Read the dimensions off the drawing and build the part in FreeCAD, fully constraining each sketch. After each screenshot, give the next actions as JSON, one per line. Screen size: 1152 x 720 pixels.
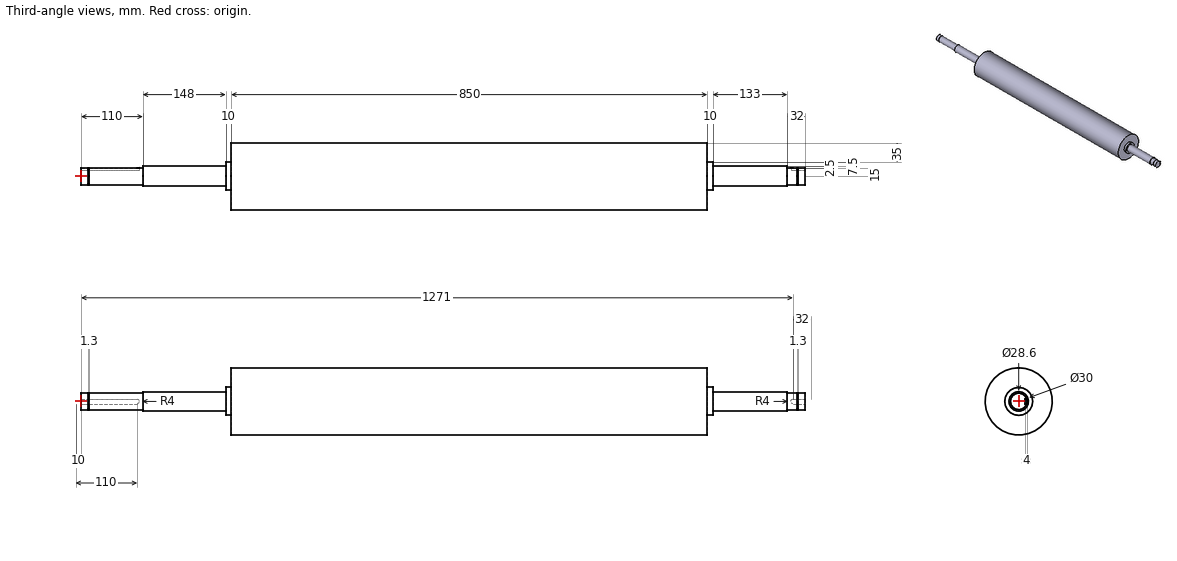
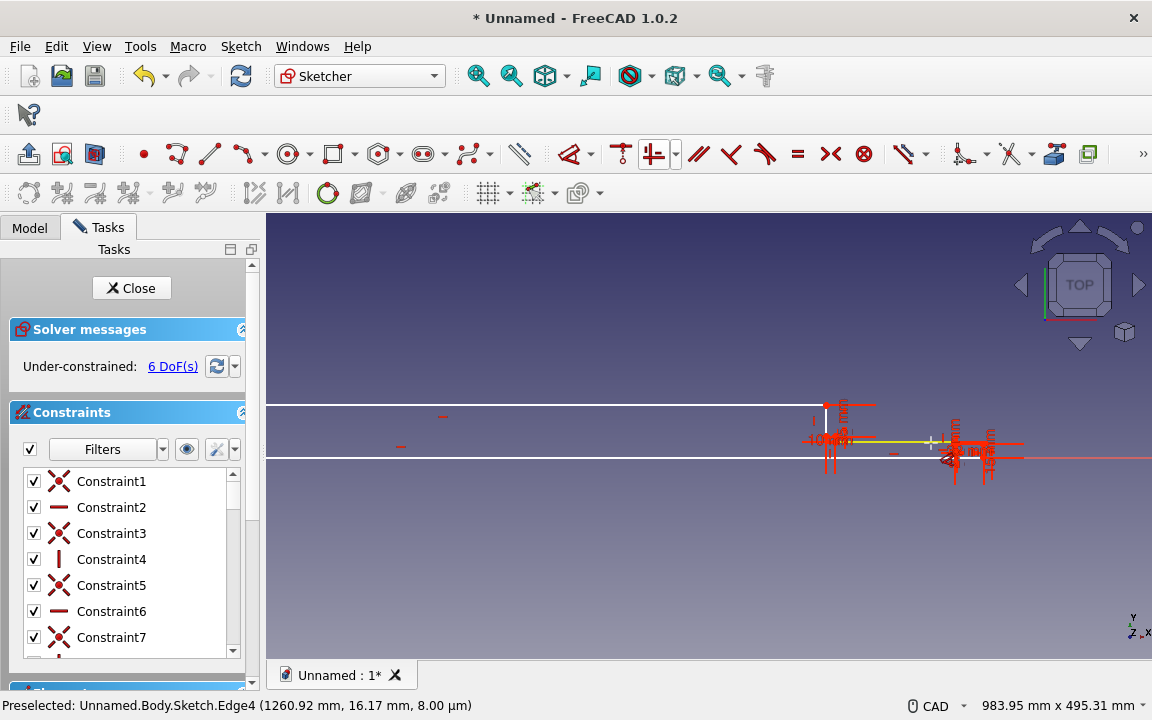
{"action": "left_click", "coordinate": [931, 442]}
{"action": "left_click", "coordinate": [895, 476]}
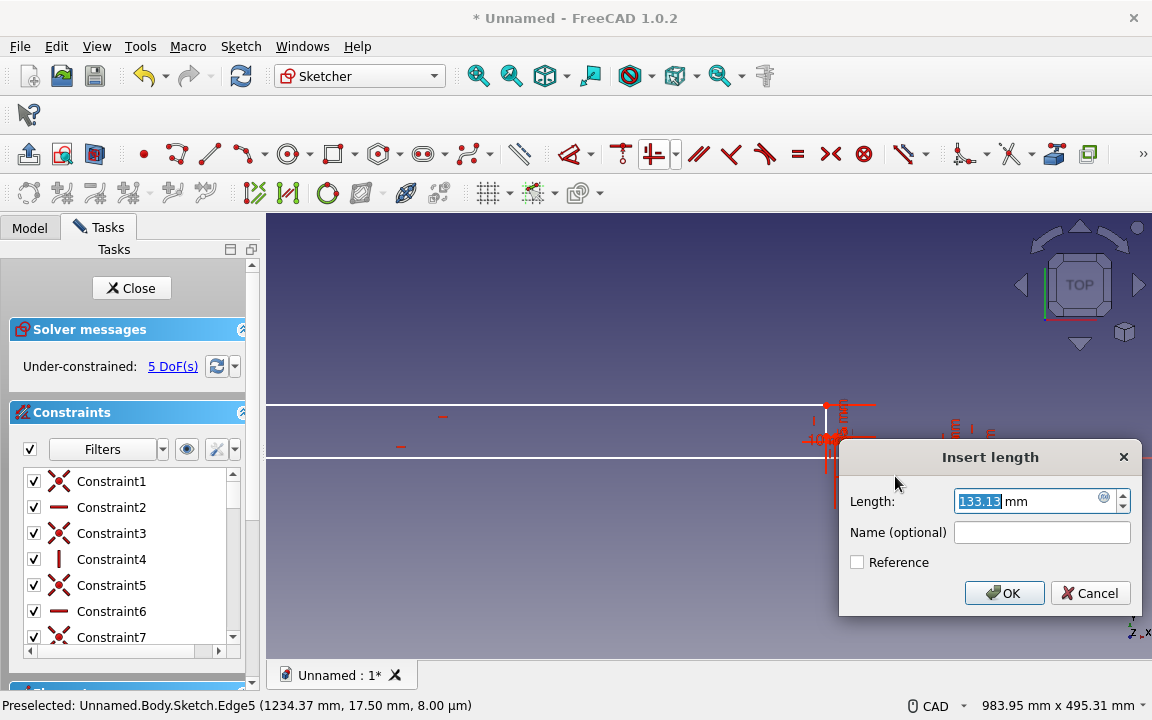
{"action": "type", "text": "133"}
{"action": "key", "text": "Return"}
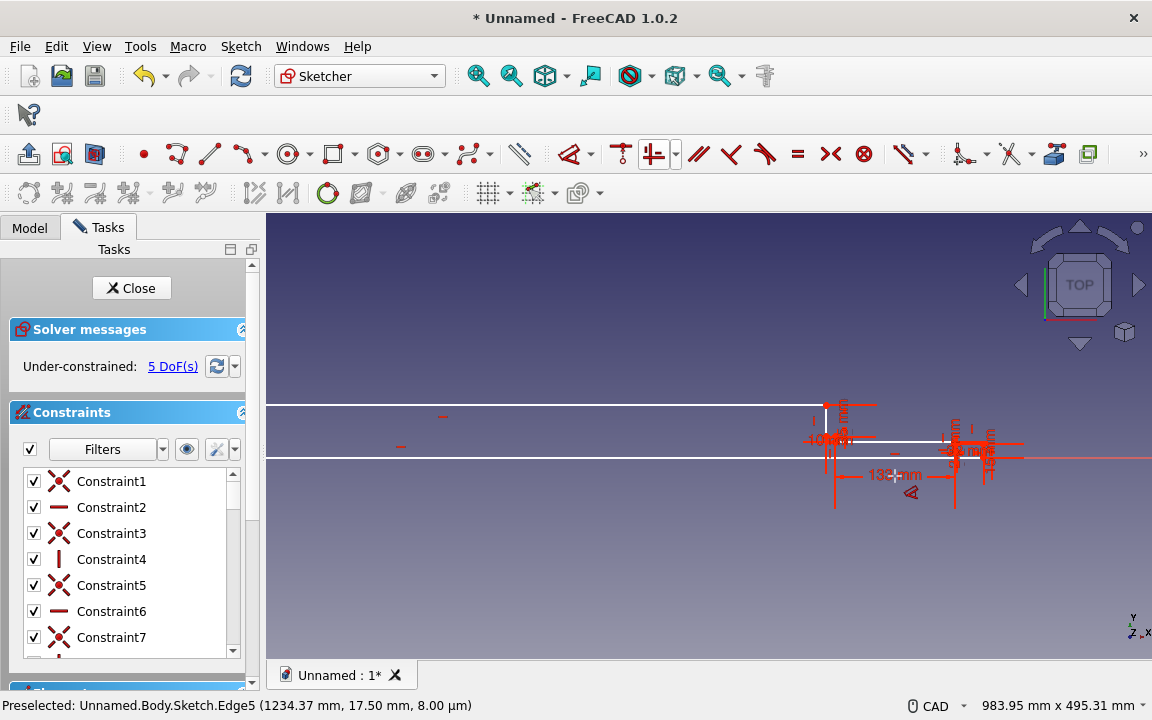
{"action": "scroll", "coordinate": [835, 439], "scroll_direction": "up", "scroll_amount": 9}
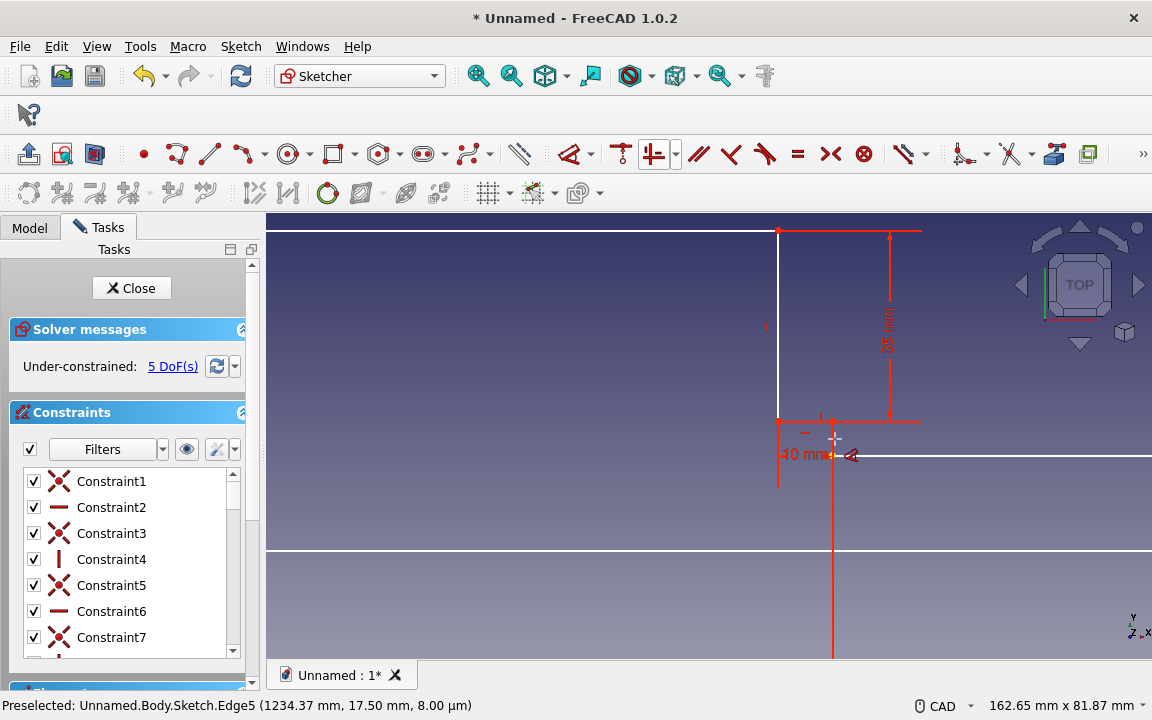
{"action": "left_click", "coordinate": [833, 439]}
{"action": "left_click", "coordinate": [867, 427]}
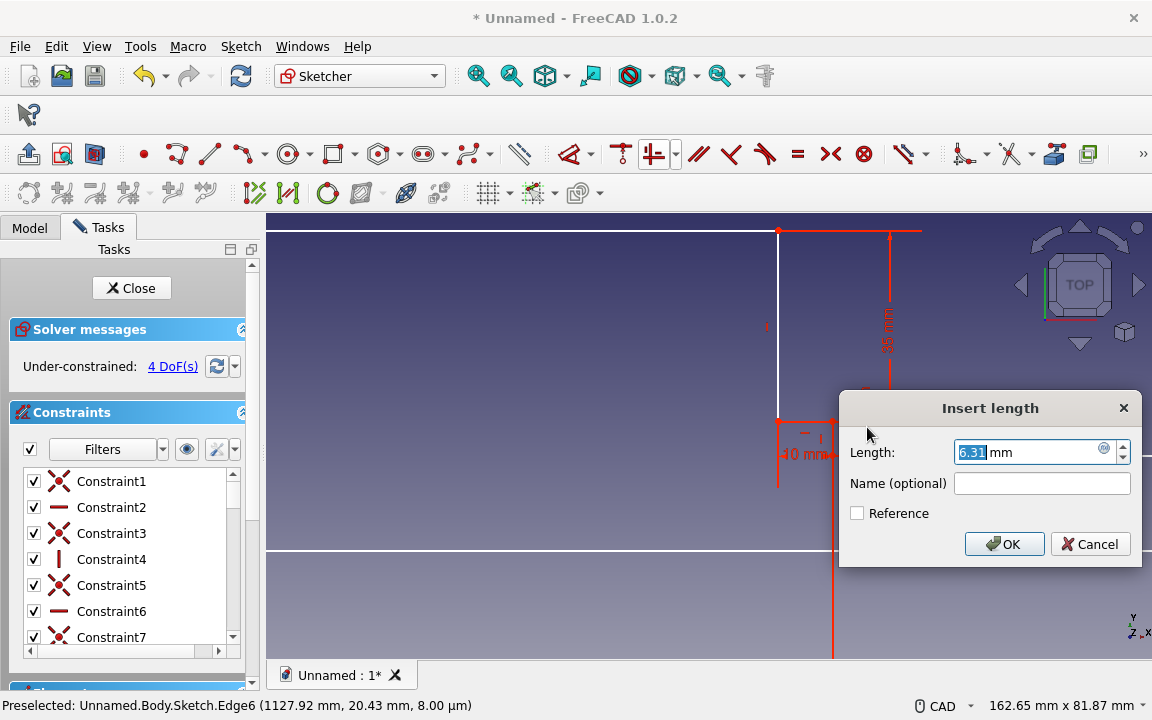
{"action": "type", "text": "7.5"}
{"action": "key", "text": "Return"}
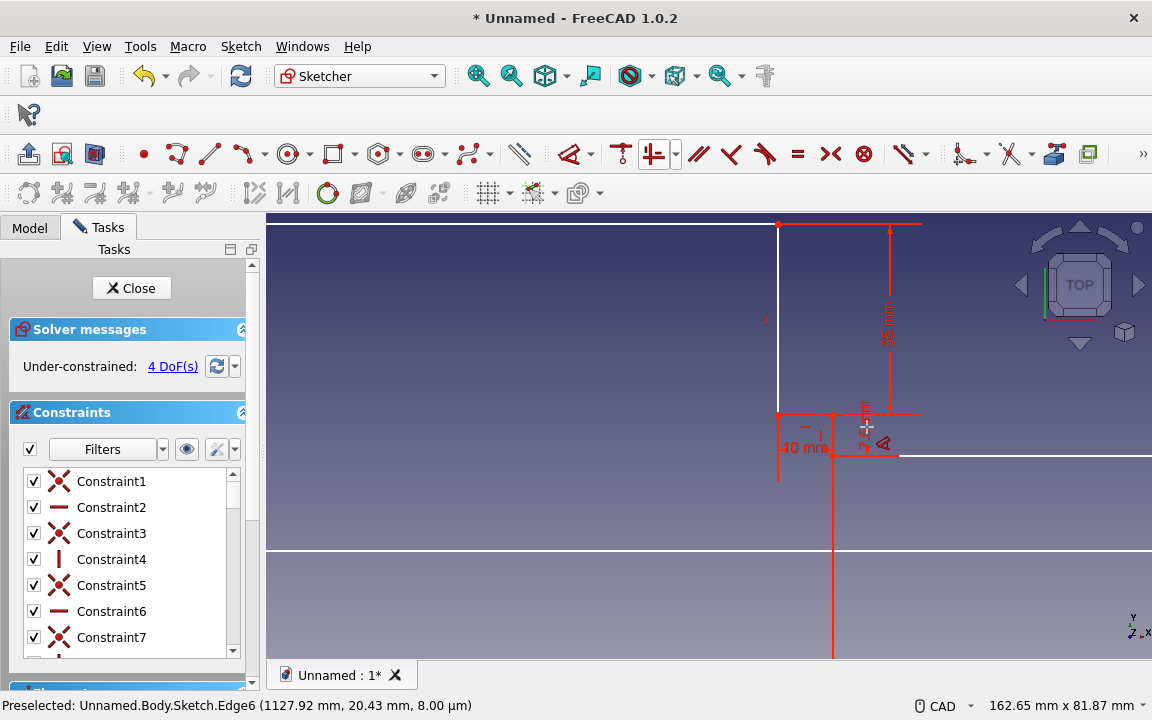
{"action": "scroll", "coordinate": [835, 440], "scroll_direction": "down", "scroll_amount": 13}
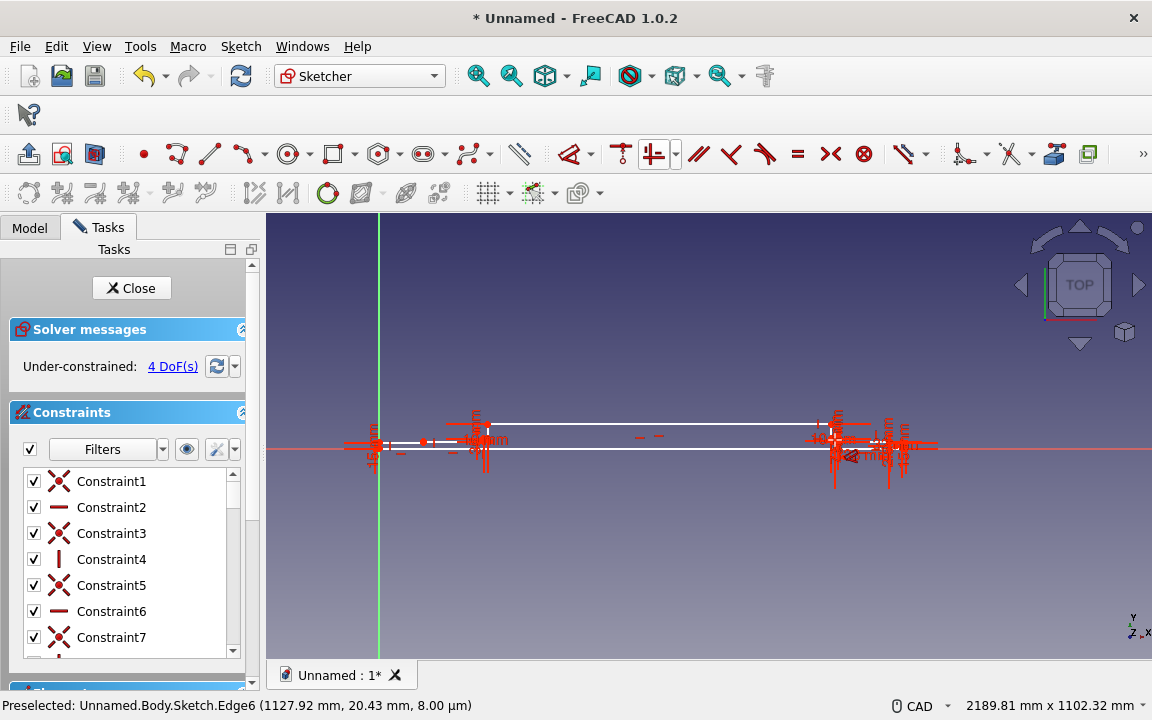
{"action": "left_click", "coordinate": [728, 424]}
{"action": "left_click", "coordinate": [660, 390]}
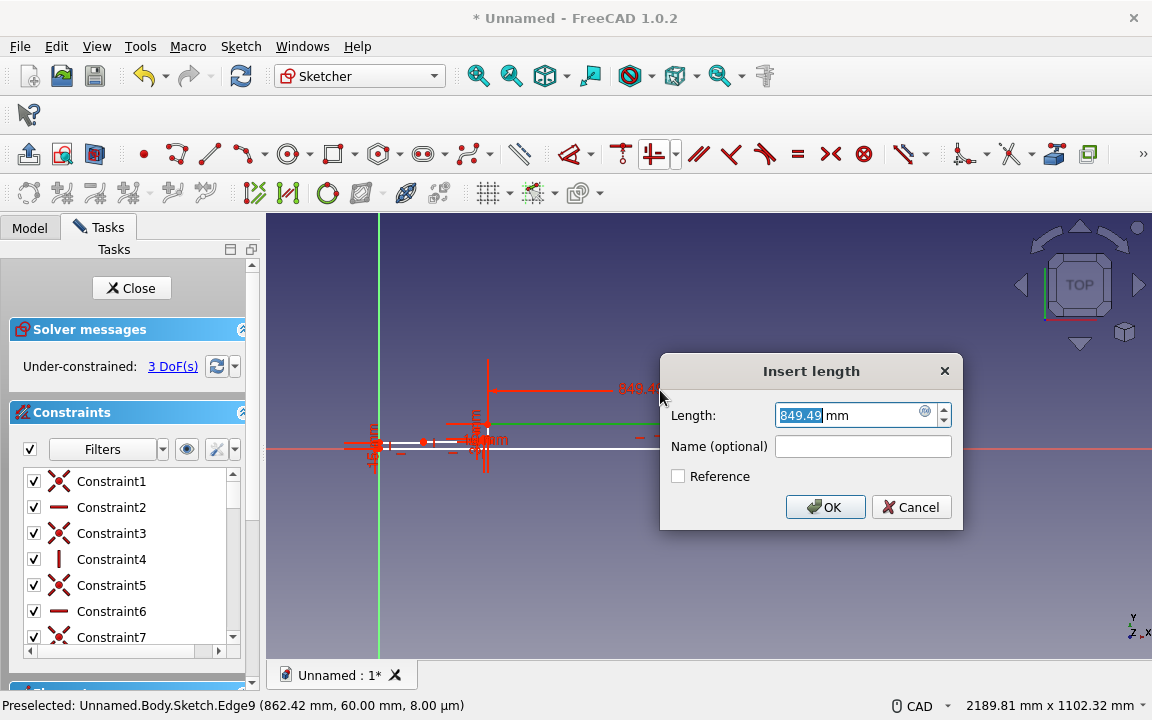
{"action": "type", "text": "850"}
{"action": "key", "text": "Return"}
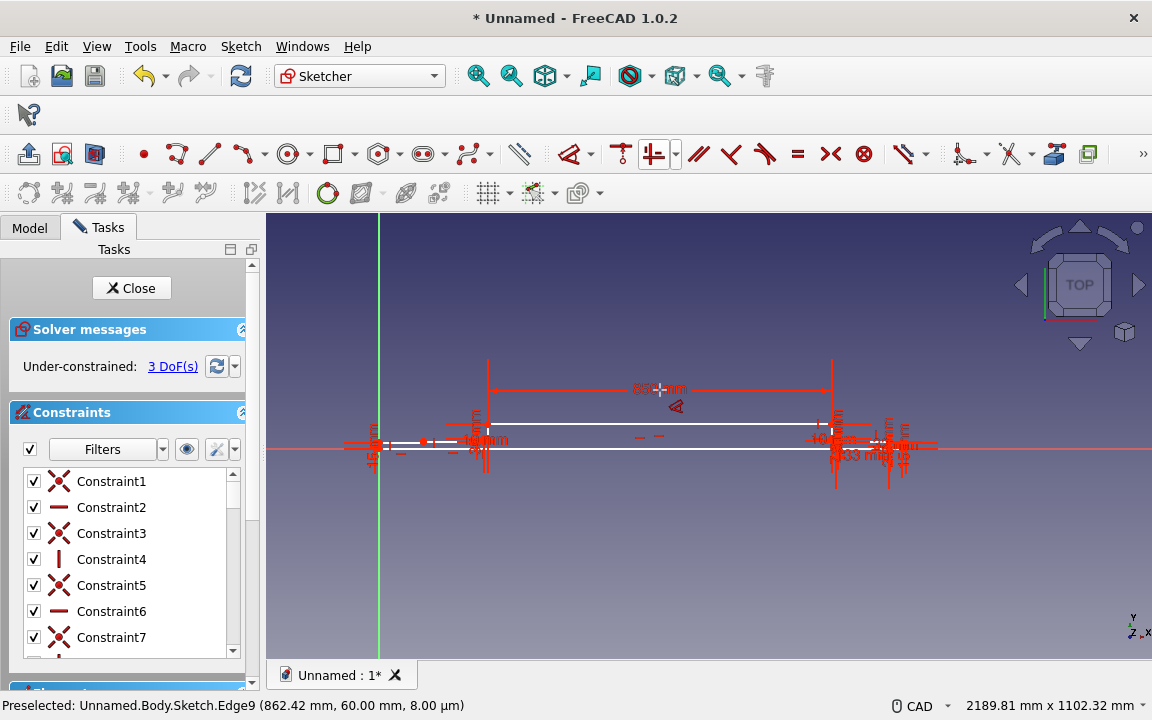
{"action": "scroll", "coordinate": [484, 440], "scroll_direction": "up", "scroll_amount": 13}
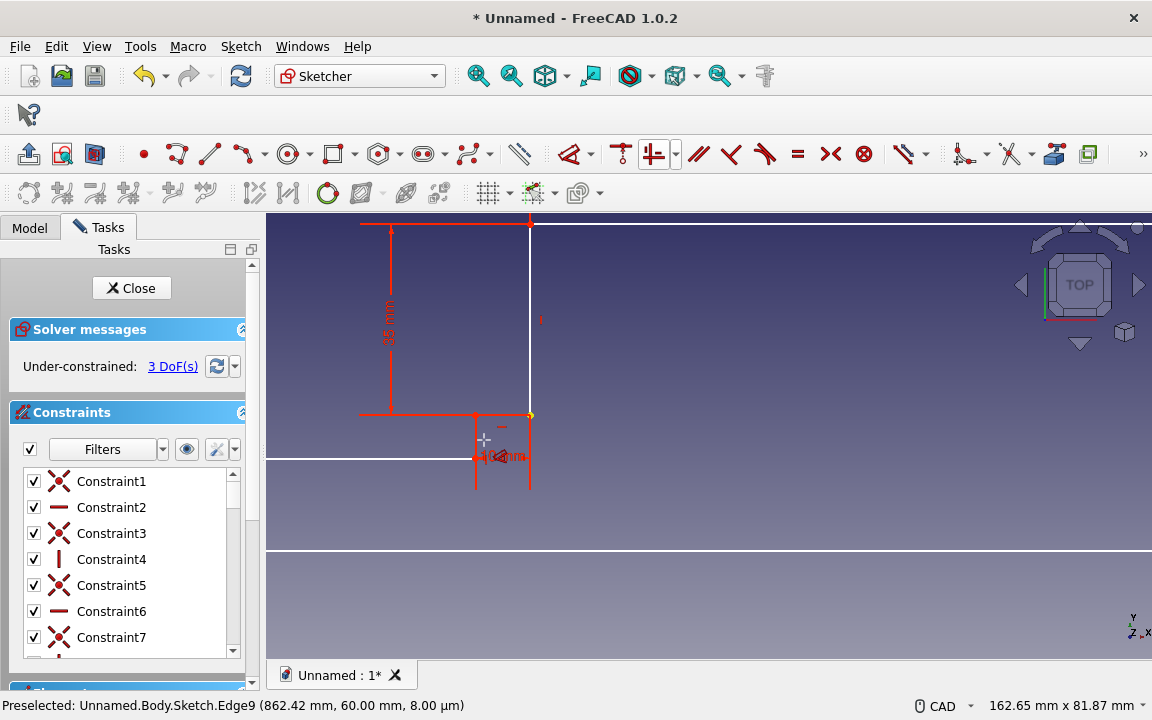
{"action": "left_click", "coordinate": [476, 437]}
{"action": "left_click", "coordinate": [442, 437]}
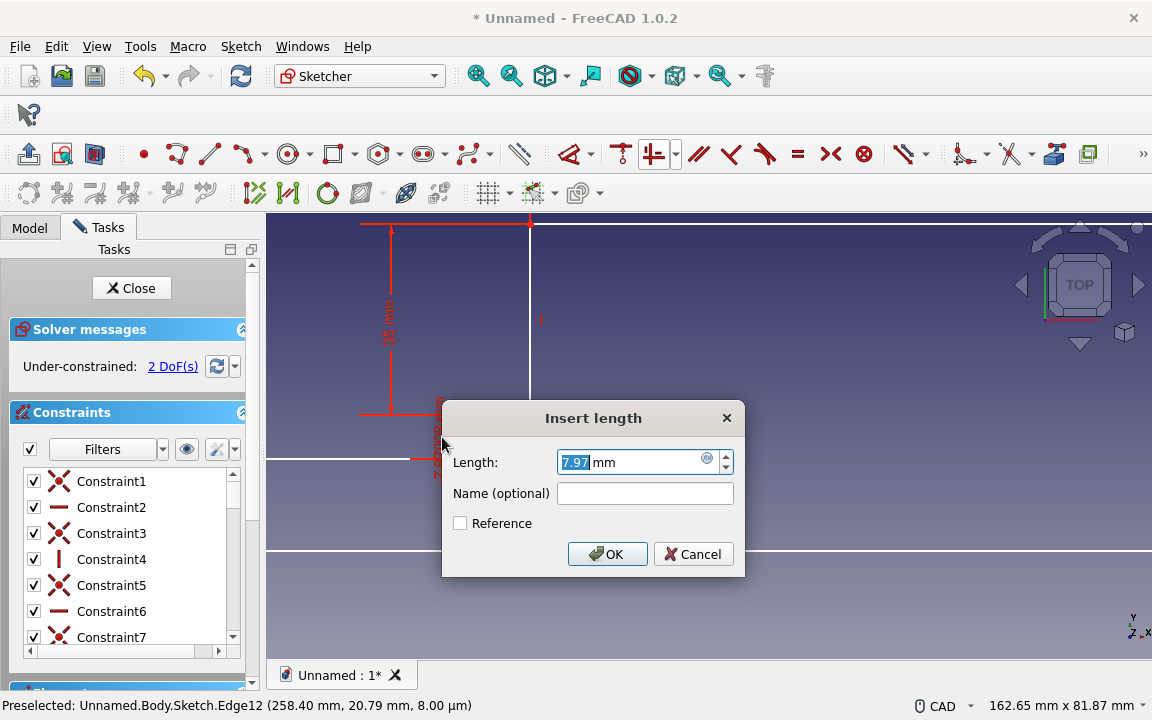
{"action": "type", "text": "7.5"}
{"action": "key", "text": "Return"}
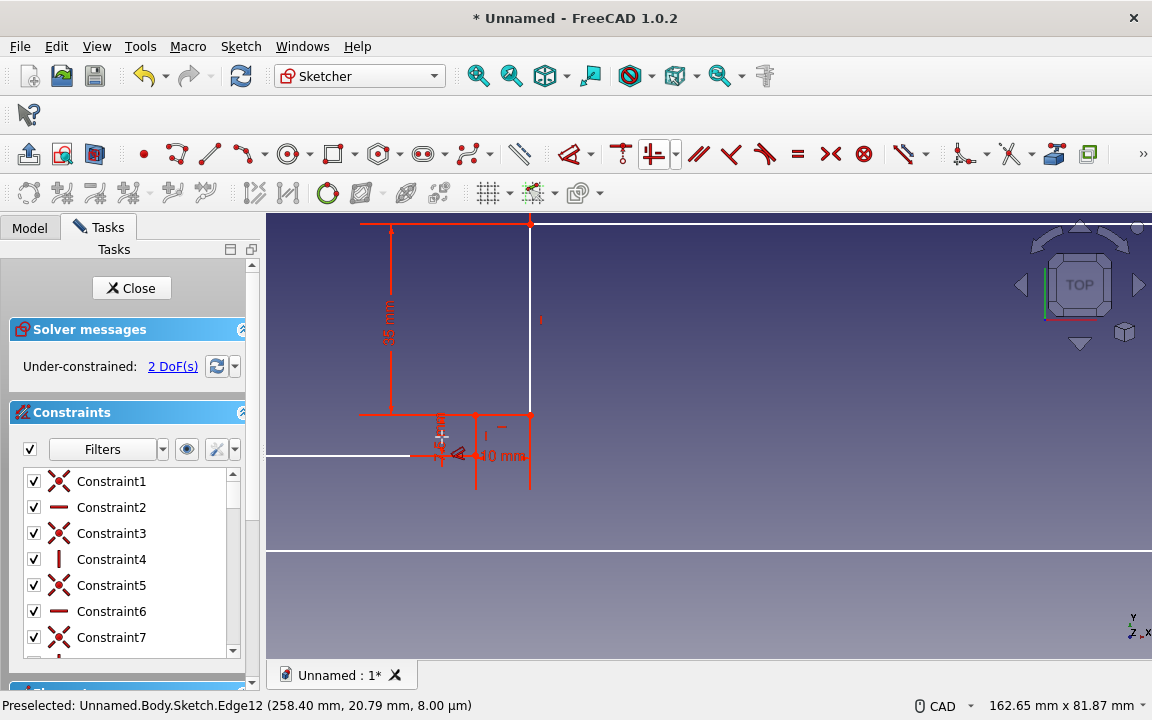
{"action": "scroll", "coordinate": [484, 440], "scroll_direction": "down", "scroll_amount": 13}